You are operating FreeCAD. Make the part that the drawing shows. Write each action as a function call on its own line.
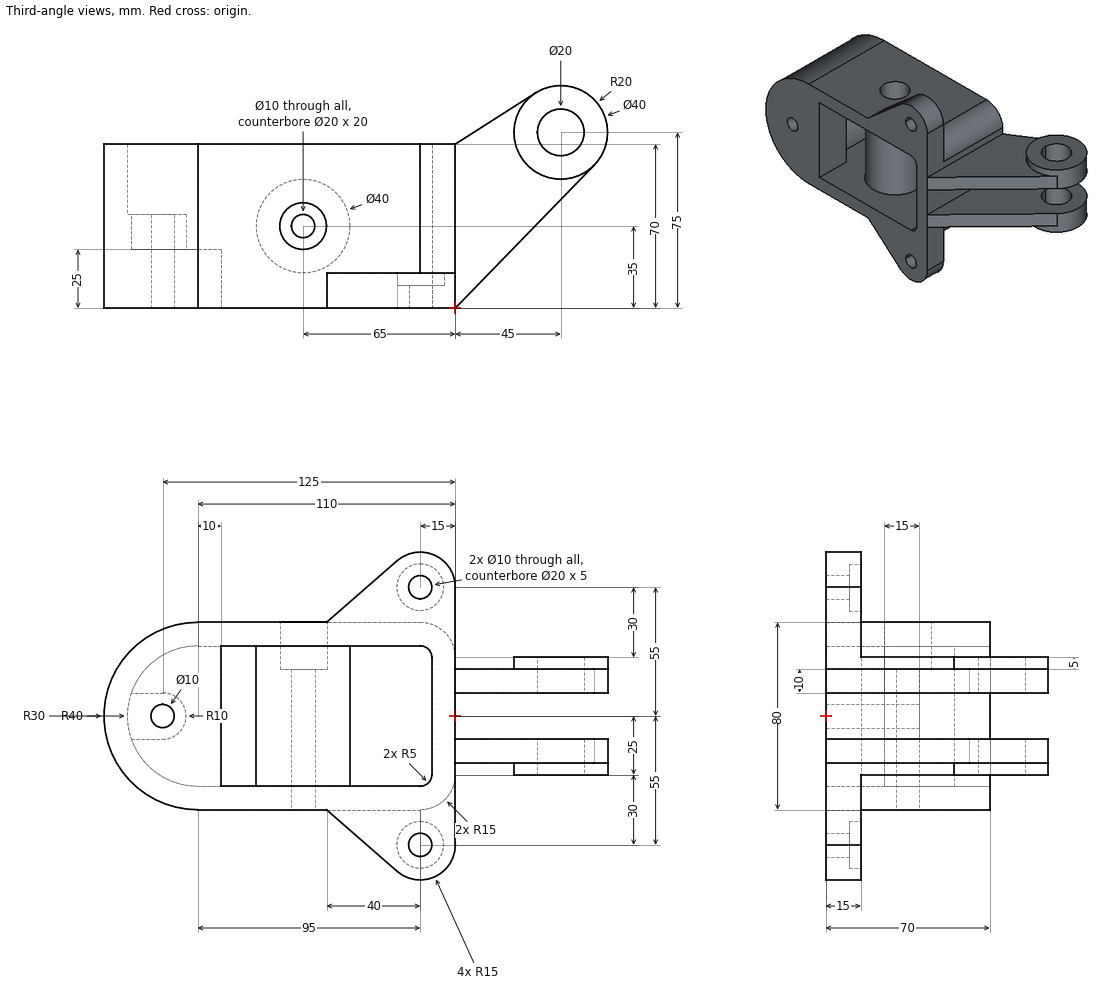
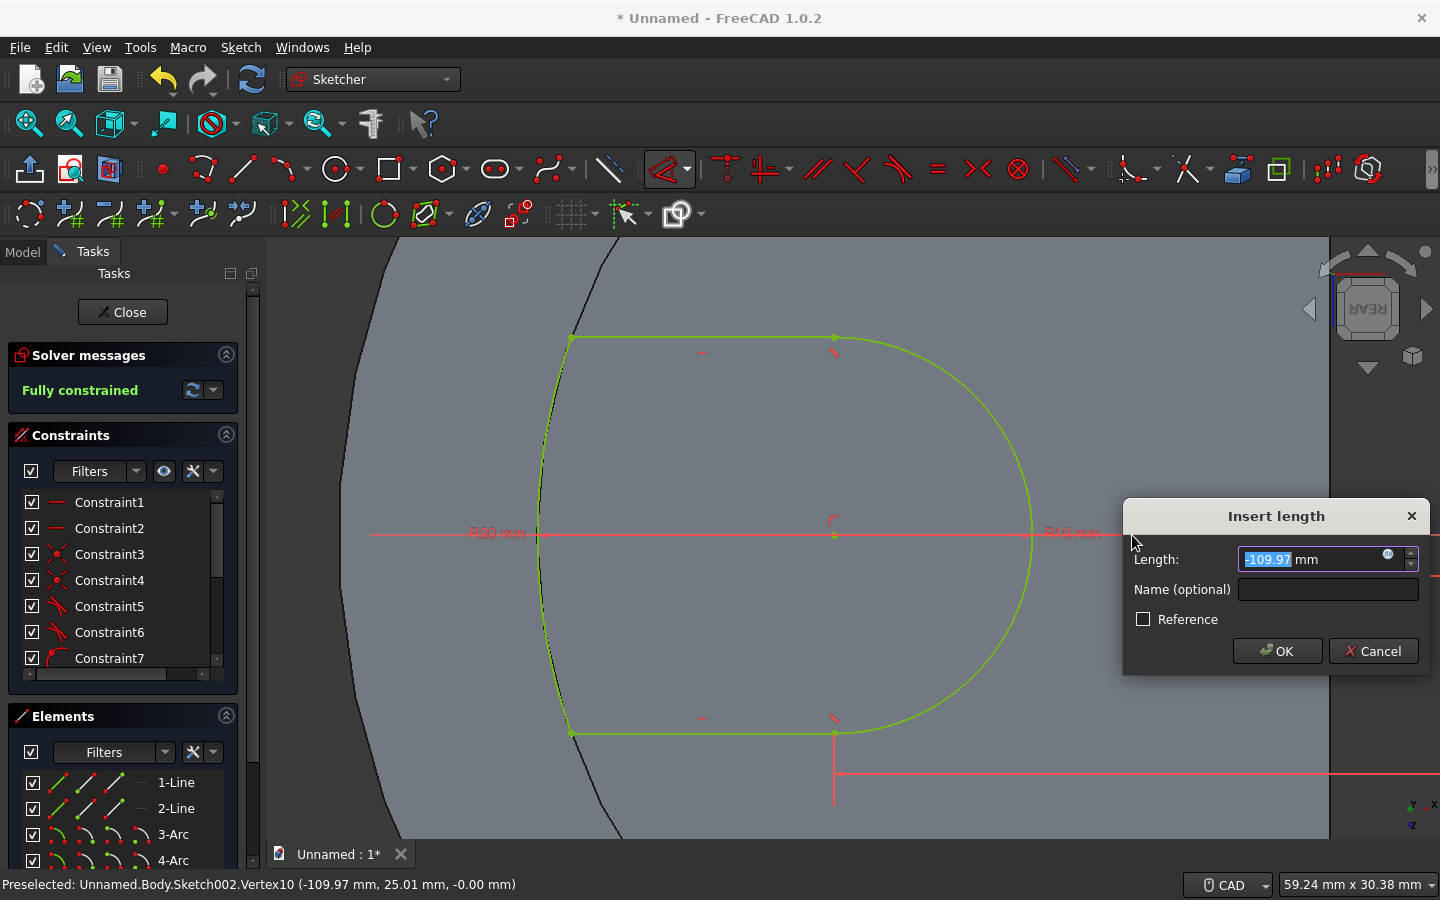
text(-110)
key(Return)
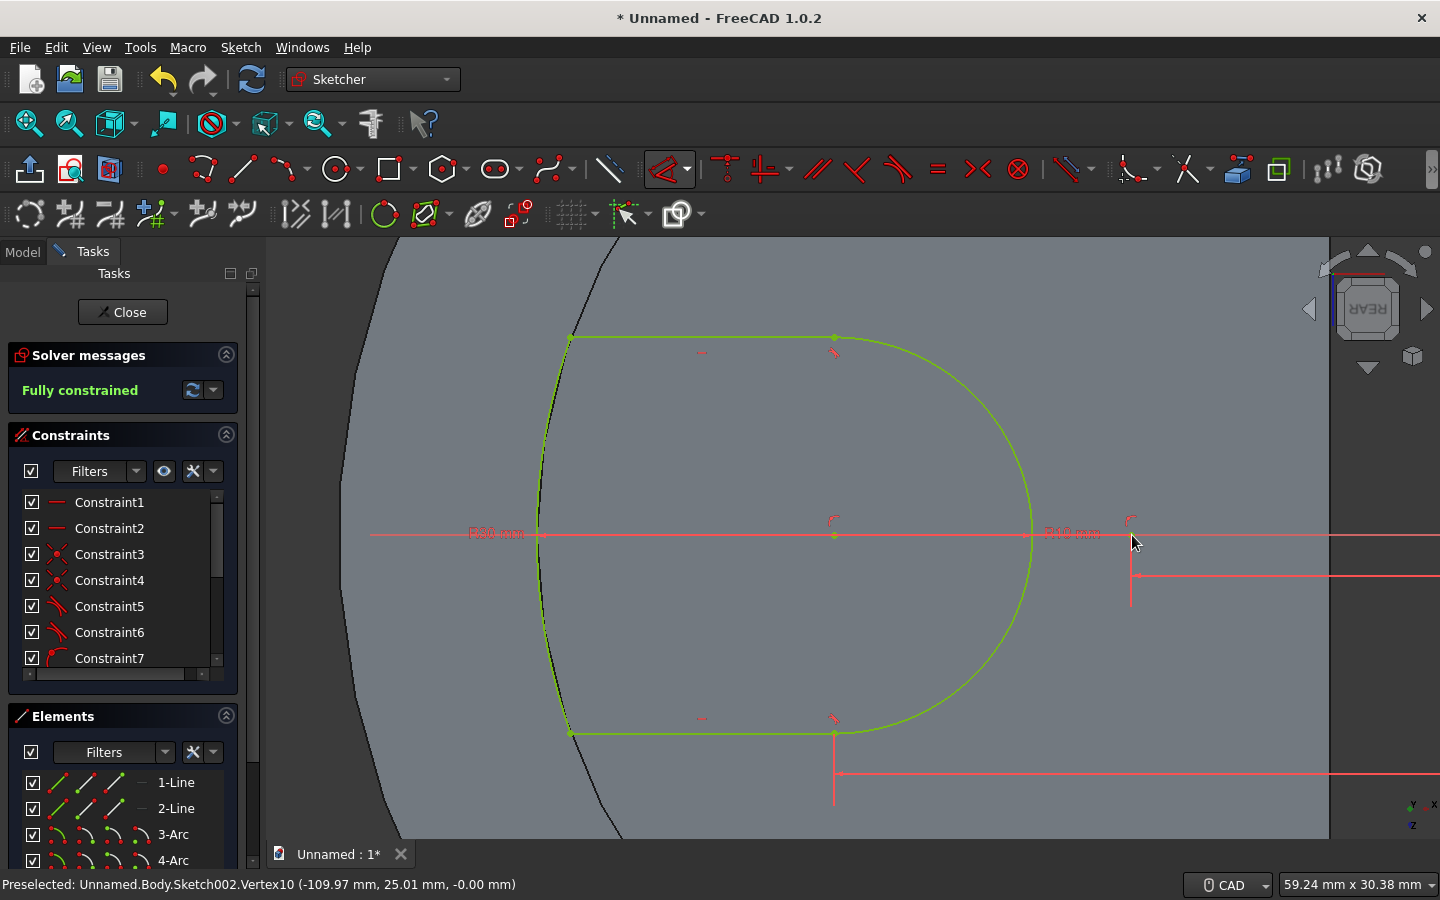
click(123, 312)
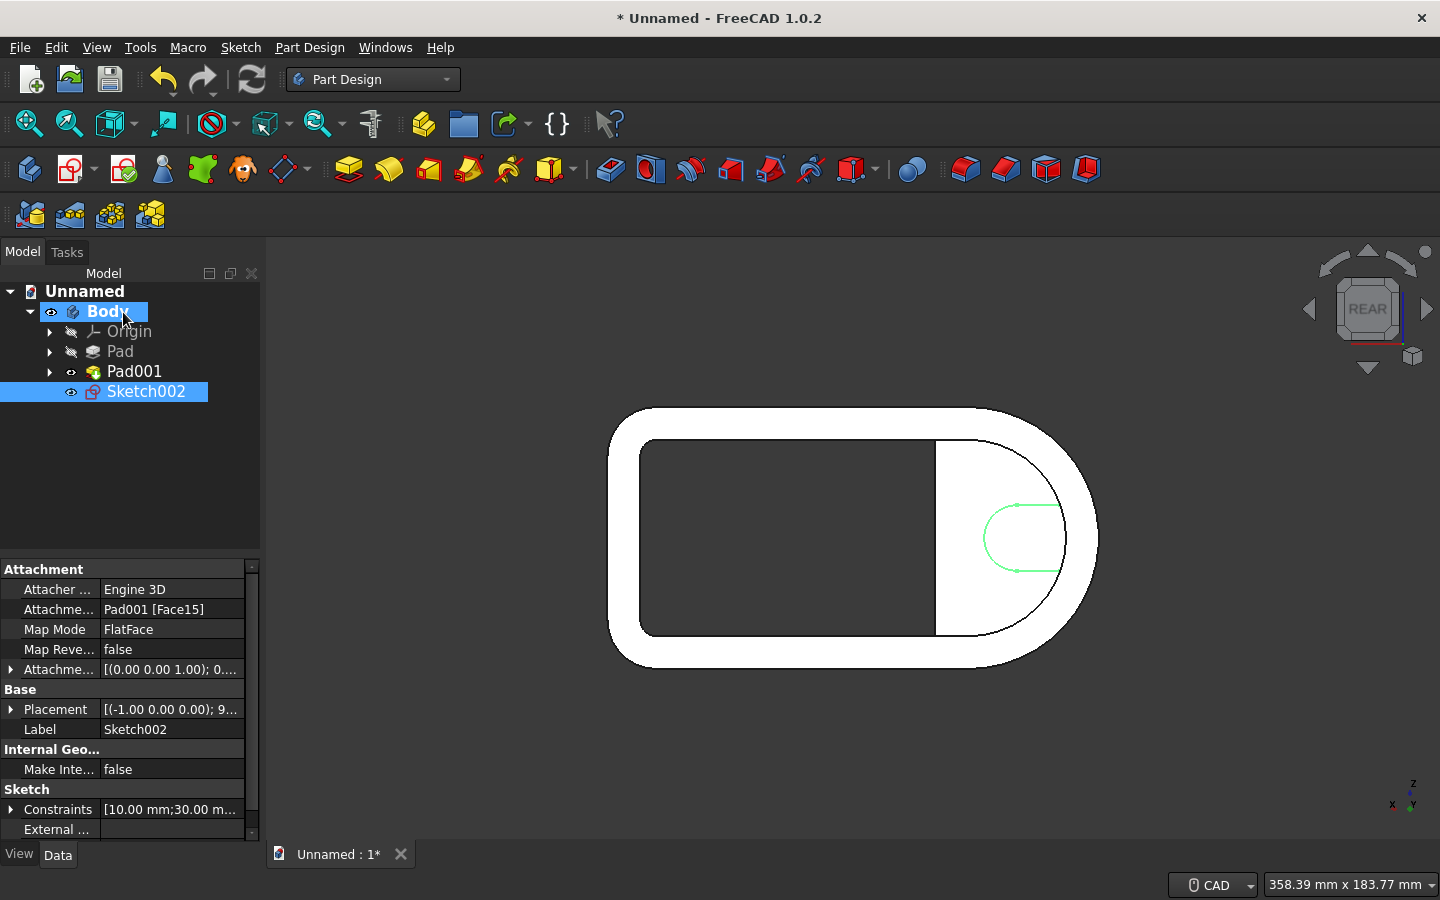
click(350, 170)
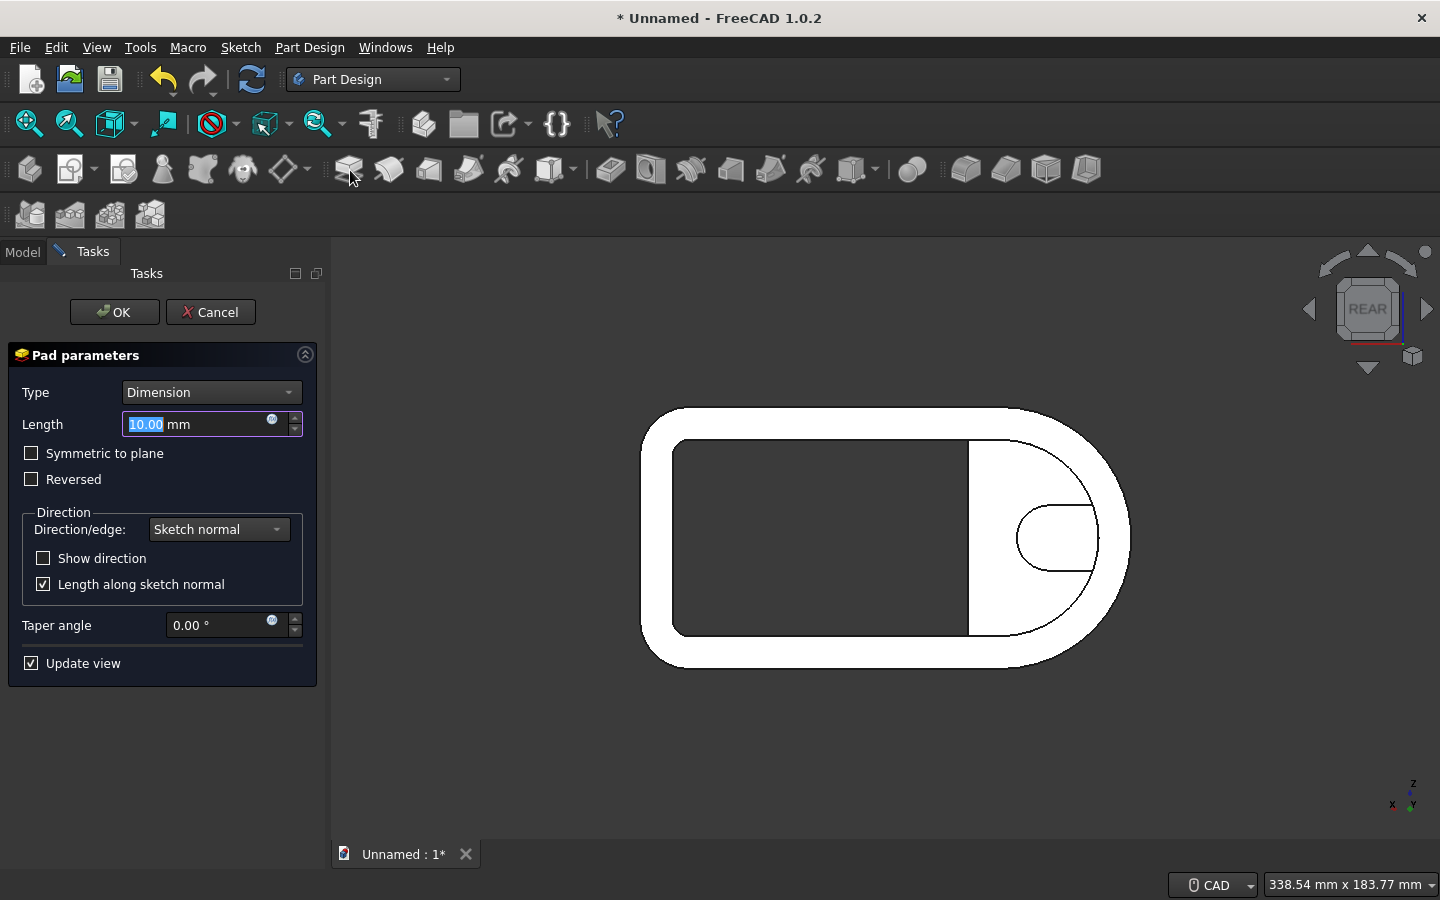
text(15)
key(Tab)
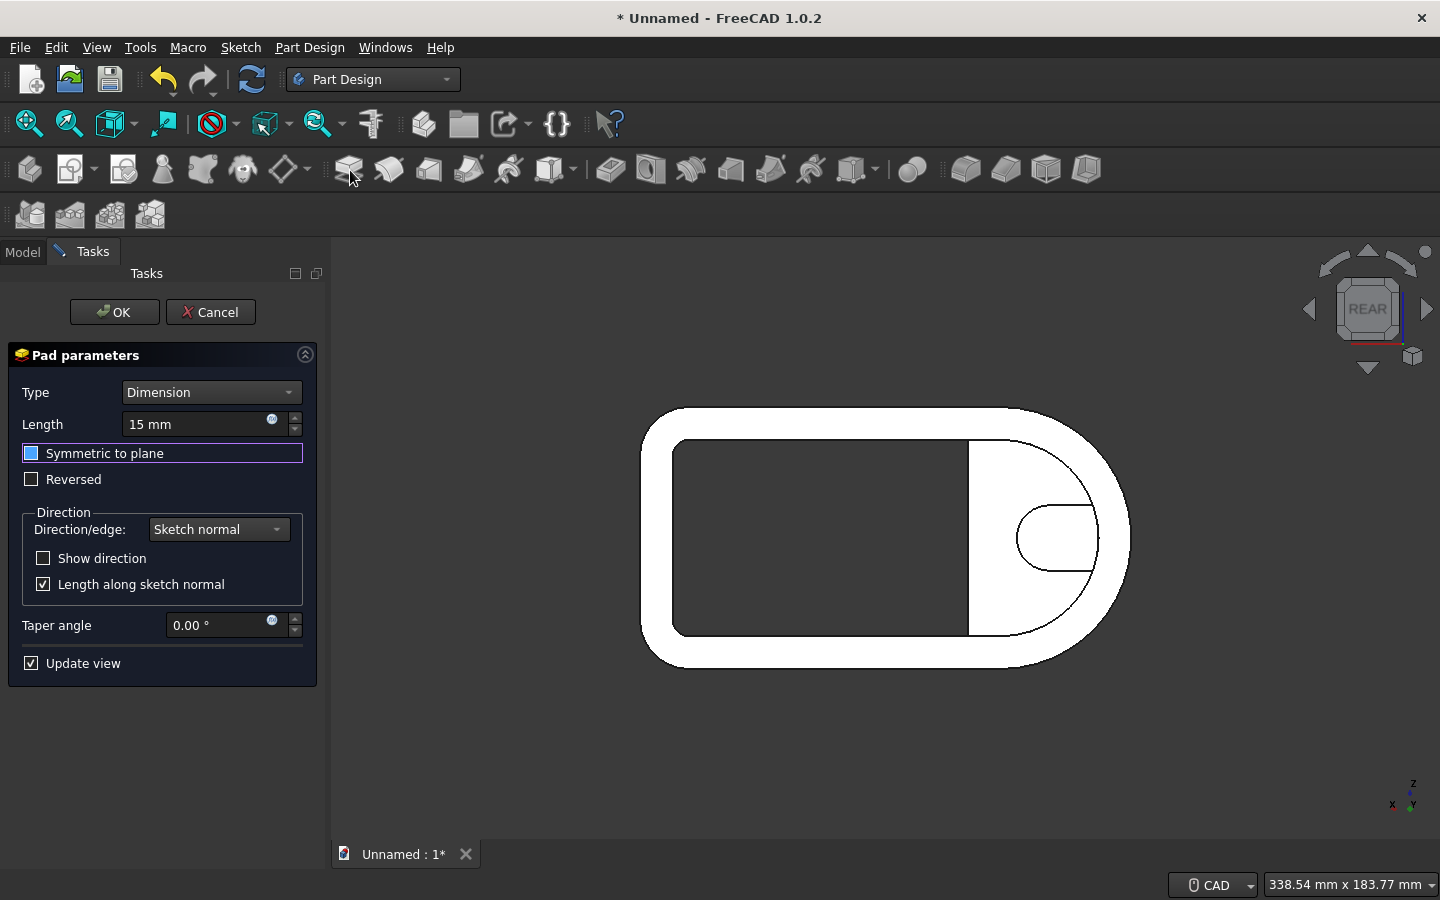
click(115, 312)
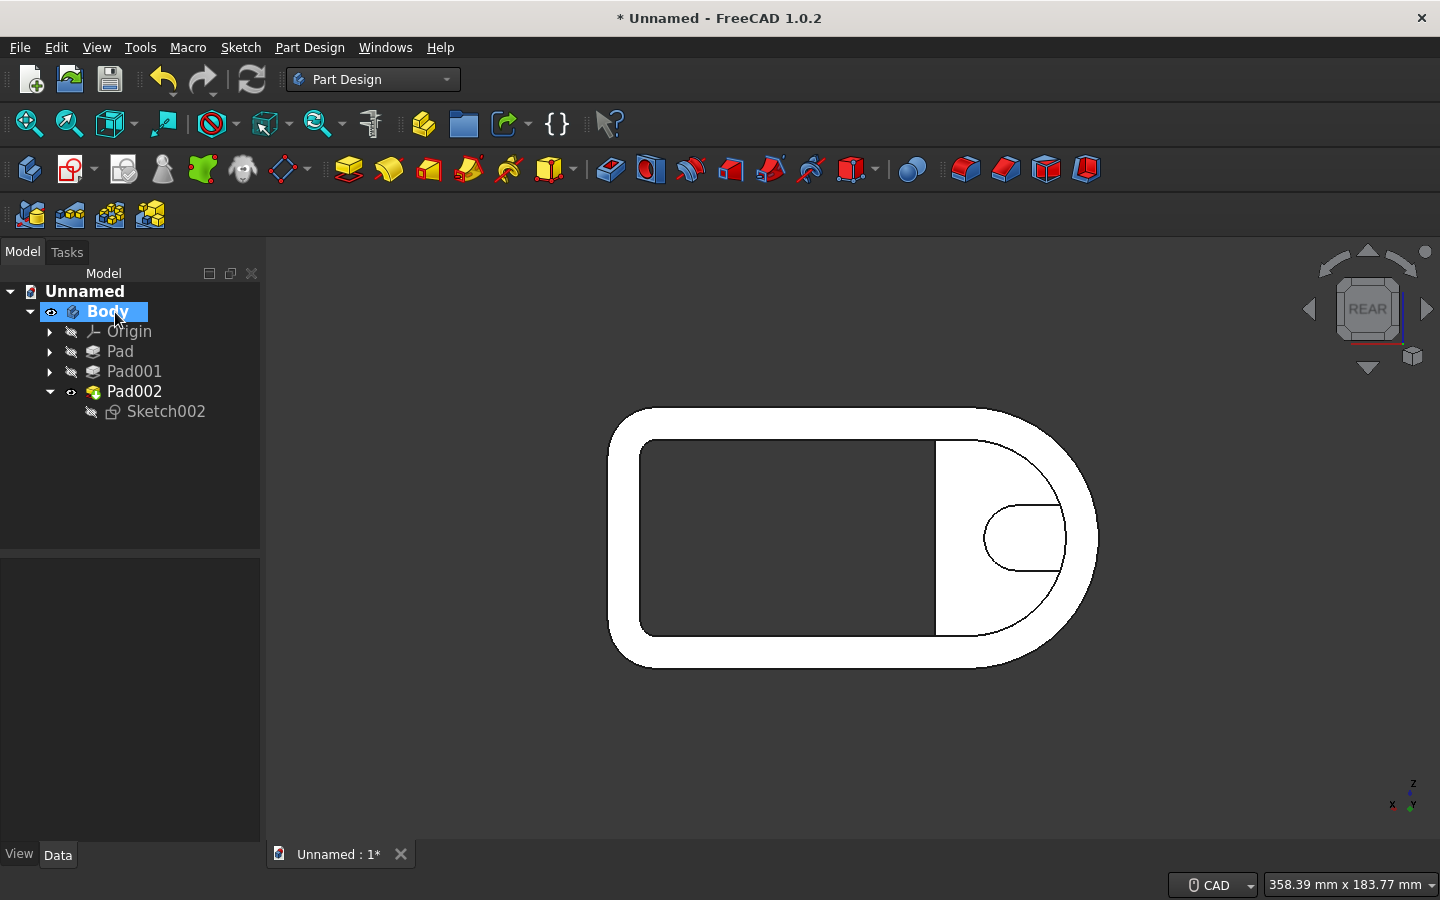
click(30, 124)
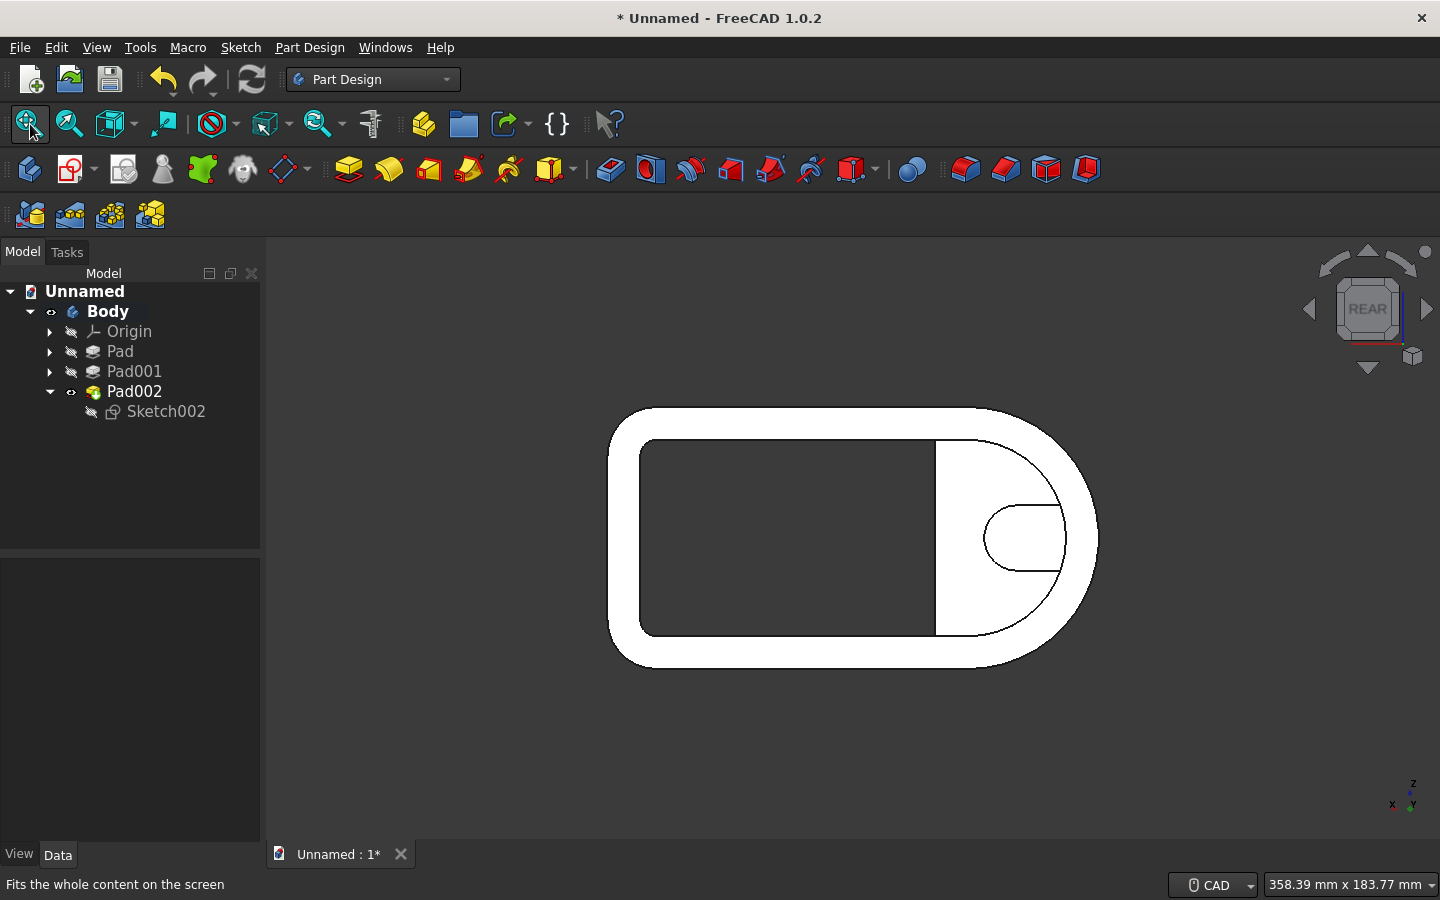
click(1025, 537)